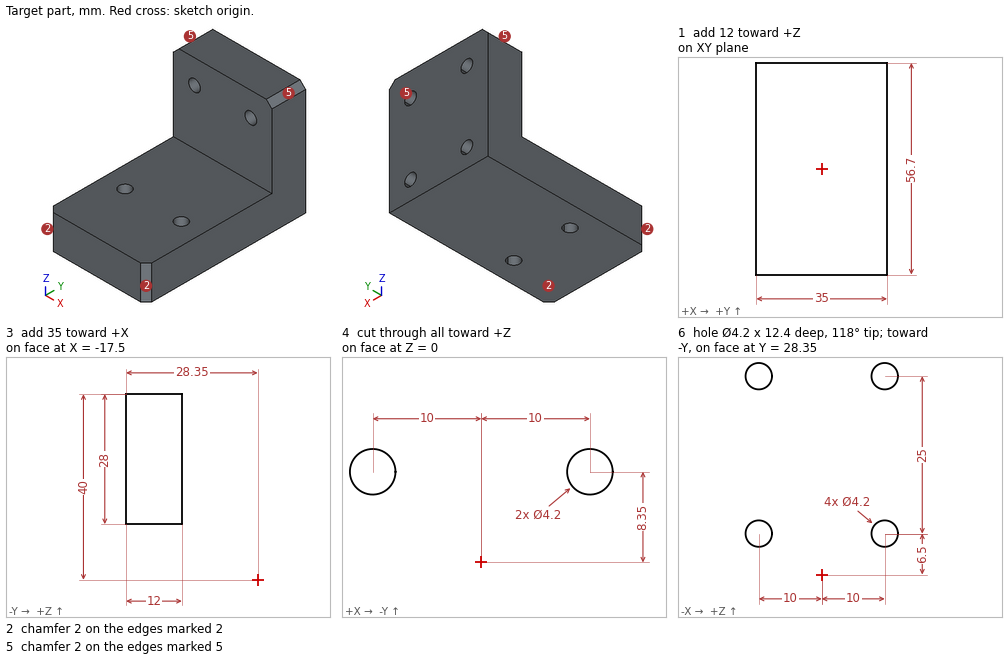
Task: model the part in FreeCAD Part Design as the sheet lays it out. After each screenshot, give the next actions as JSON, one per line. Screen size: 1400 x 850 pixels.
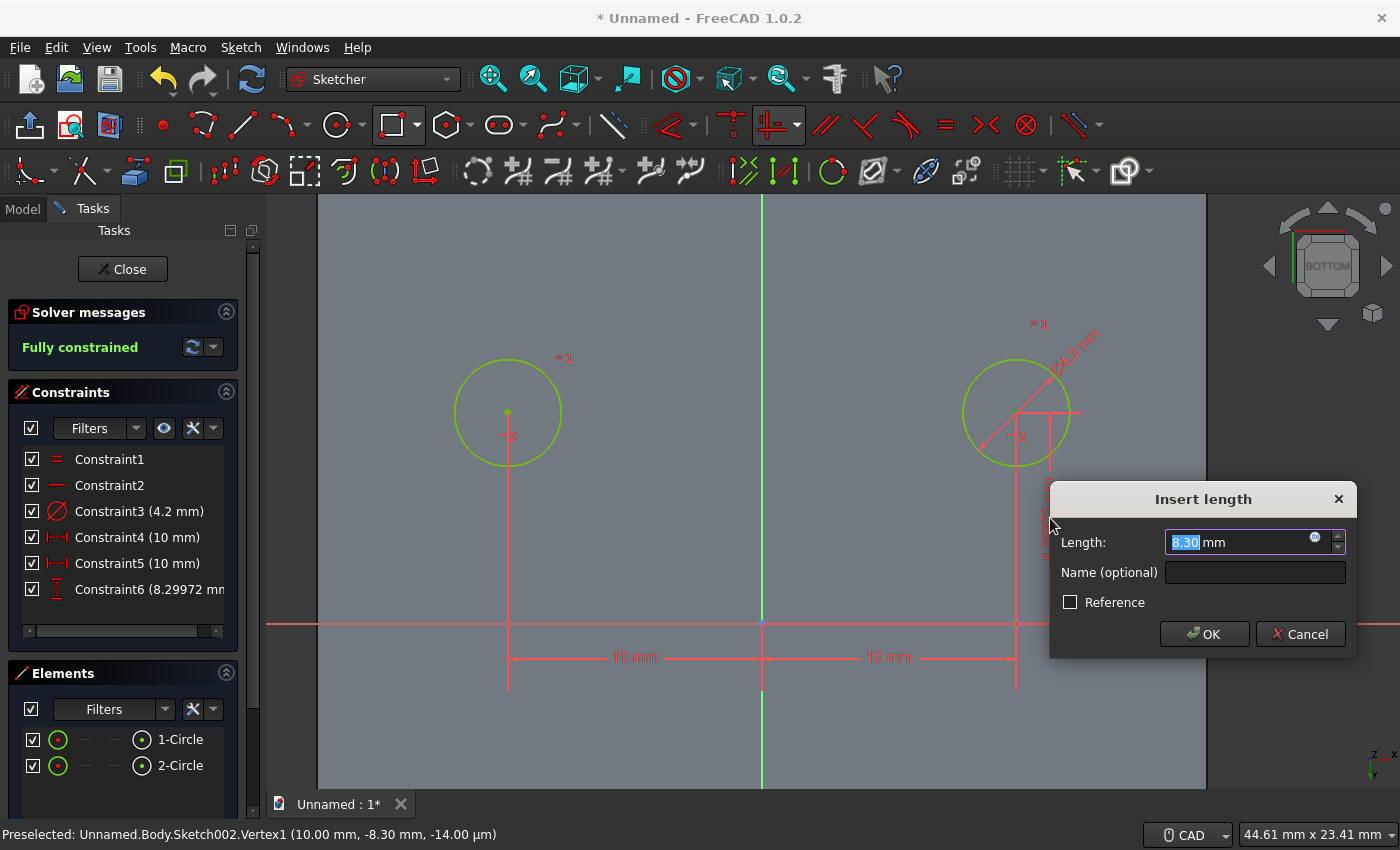
{"action": "type", "text": "8.35"}
{"action": "key", "text": "Return"}
{"action": "key", "text": "Escape"}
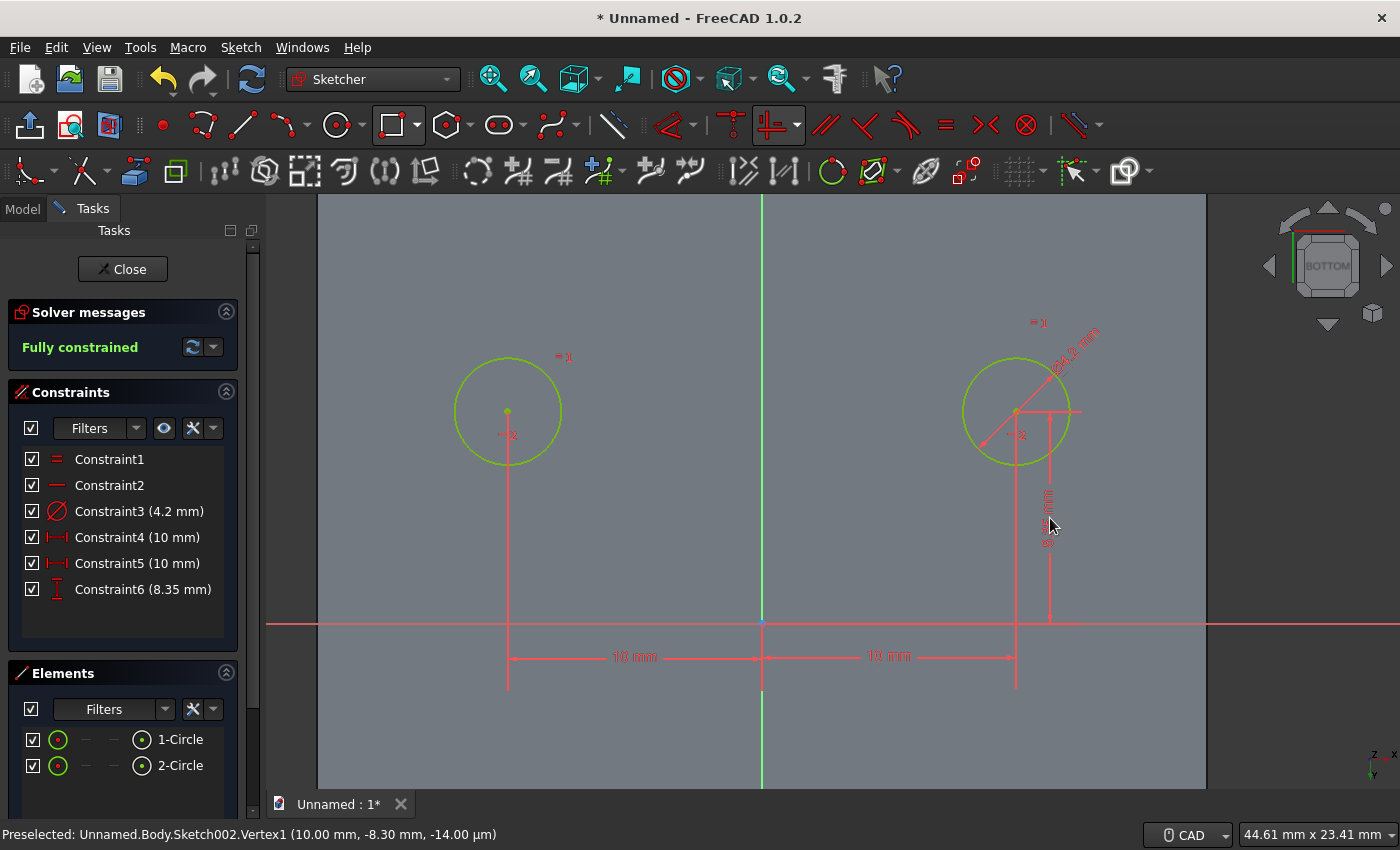
{"action": "left_click", "coordinate": [123, 269]}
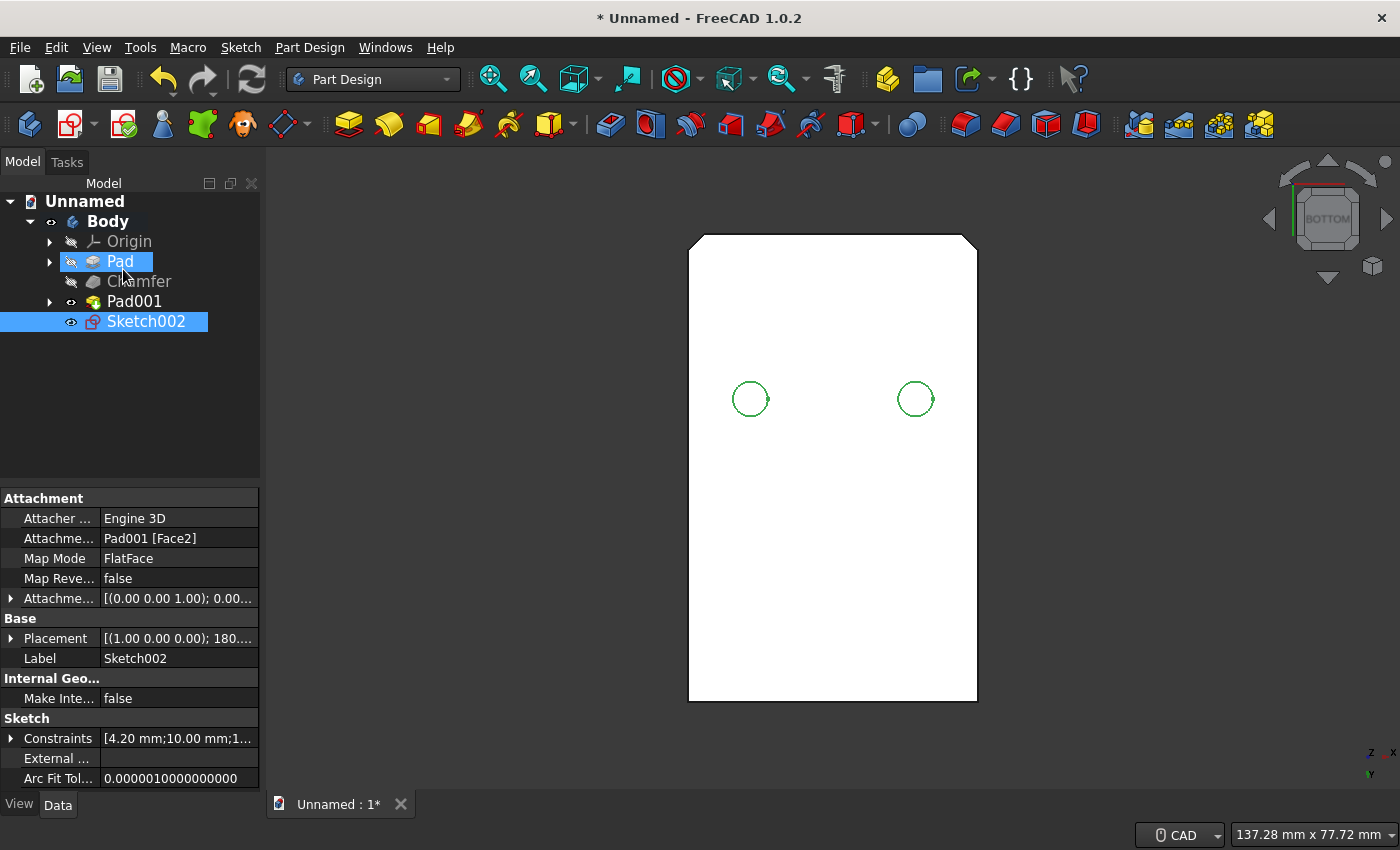
{"action": "left_click", "coordinate": [612, 124]}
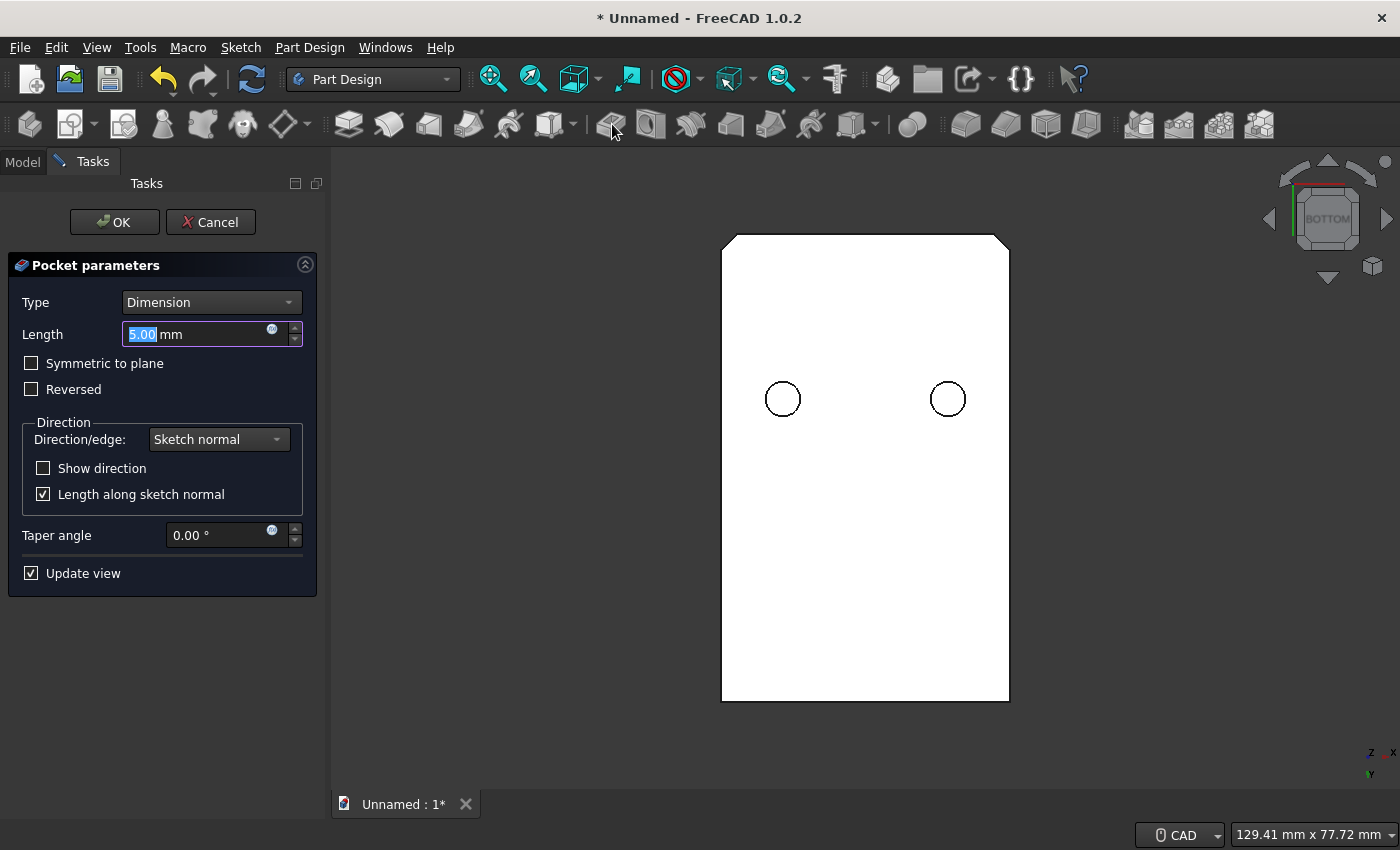
{"action": "left_click", "coordinate": [212, 302]}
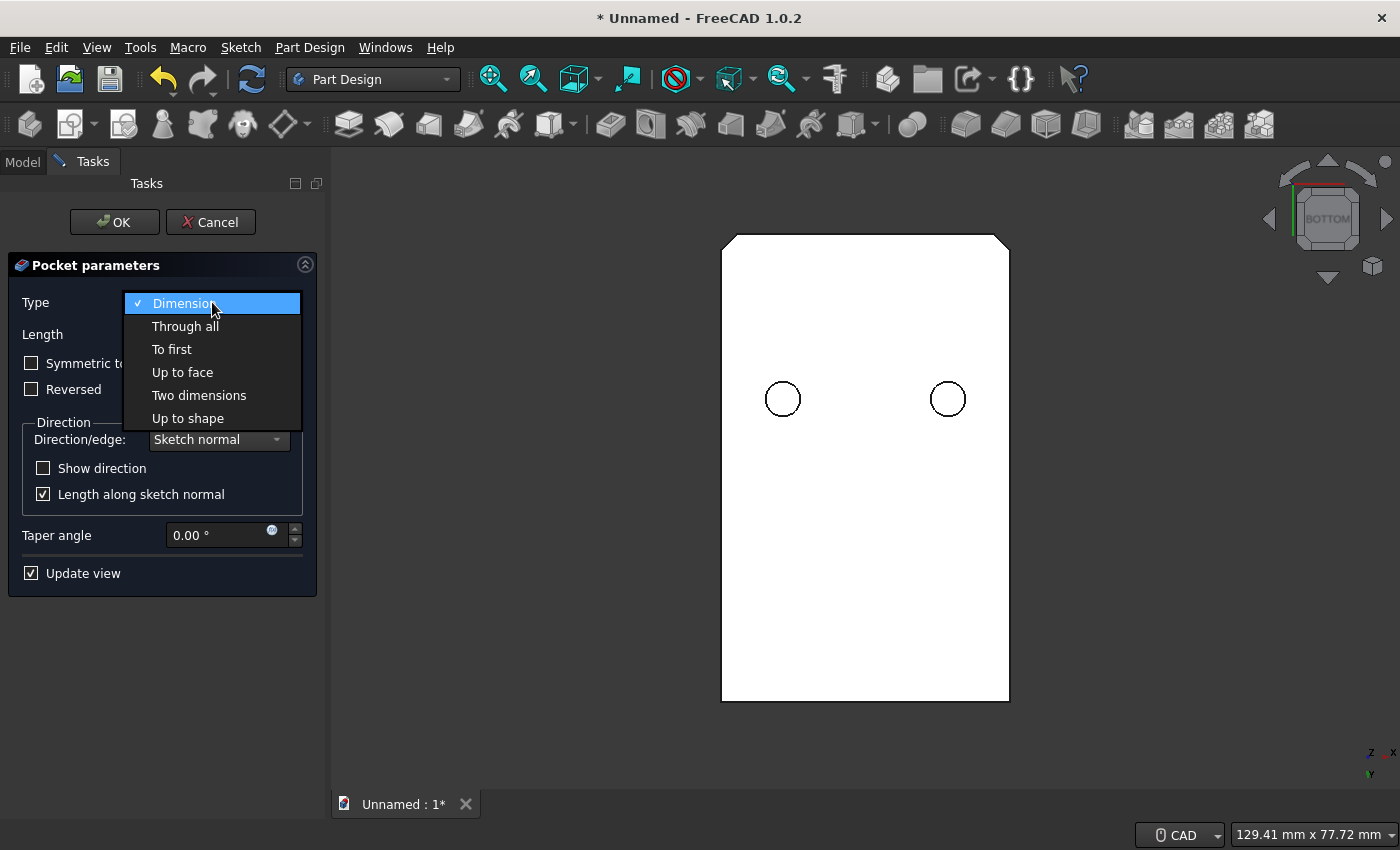
{"action": "left_click", "coordinate": [212, 326]}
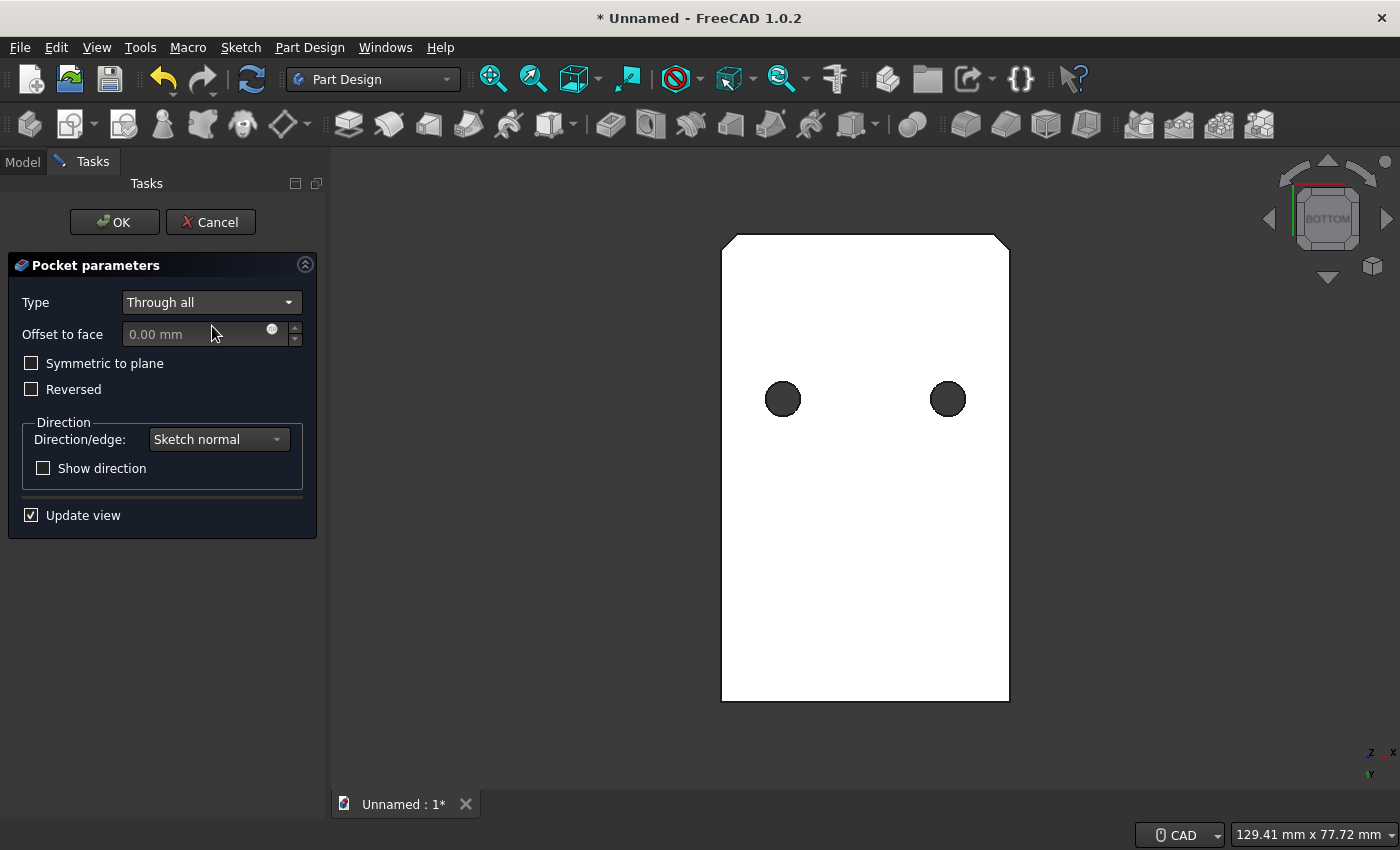
{"action": "left_click", "coordinate": [115, 222]}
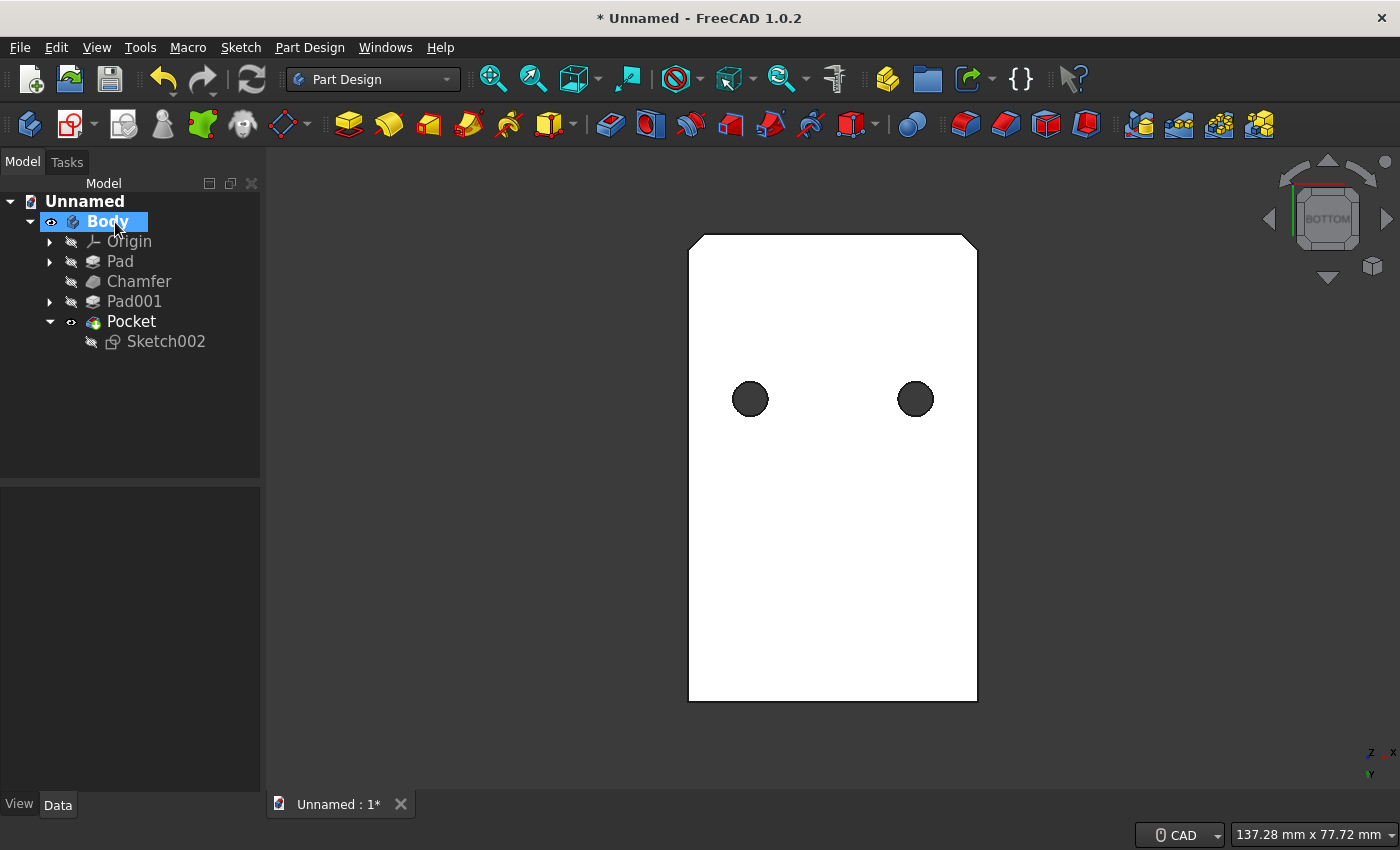
{"action": "key", "text": "0"}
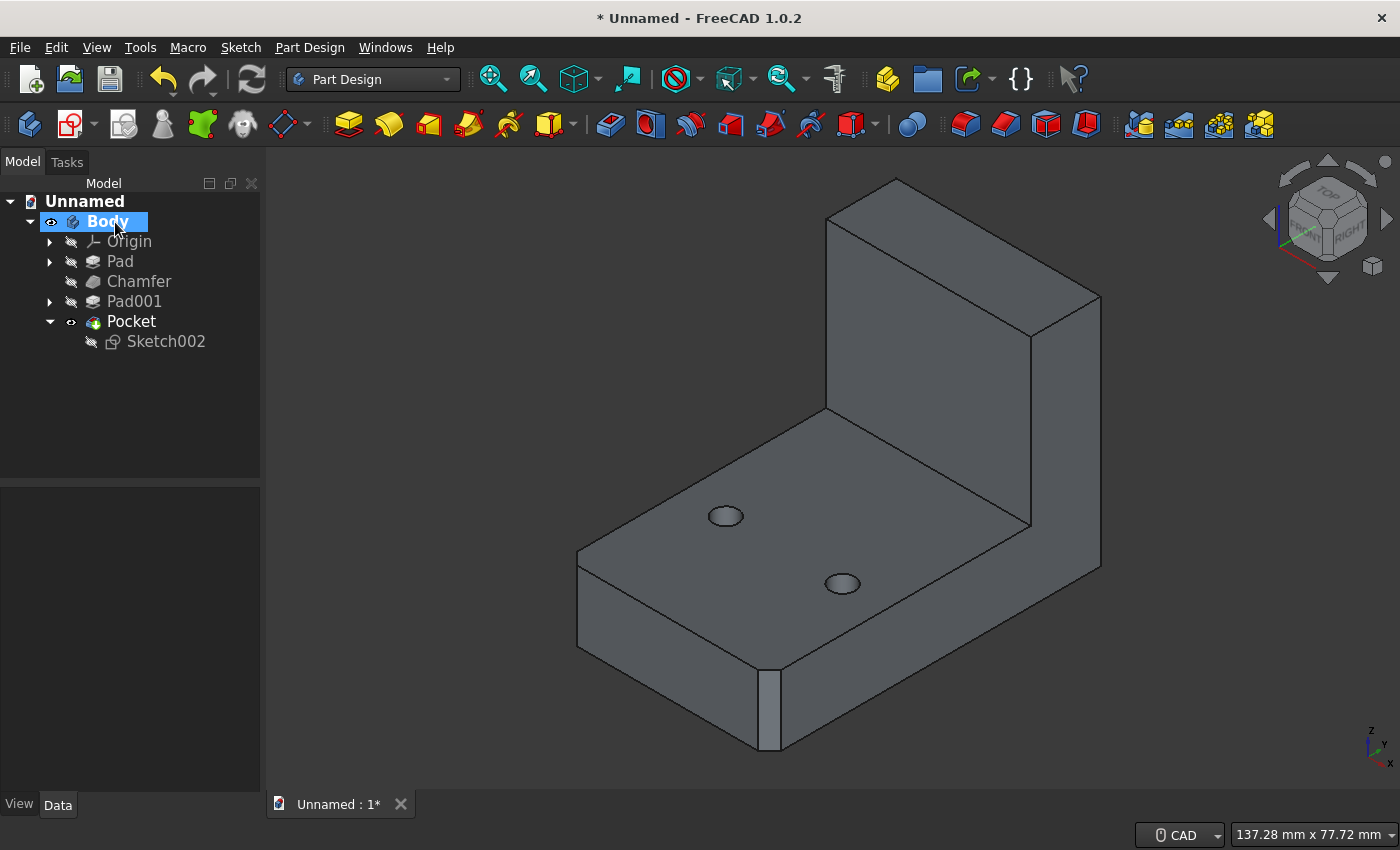
{"action": "left_click", "coordinate": [1066, 316]}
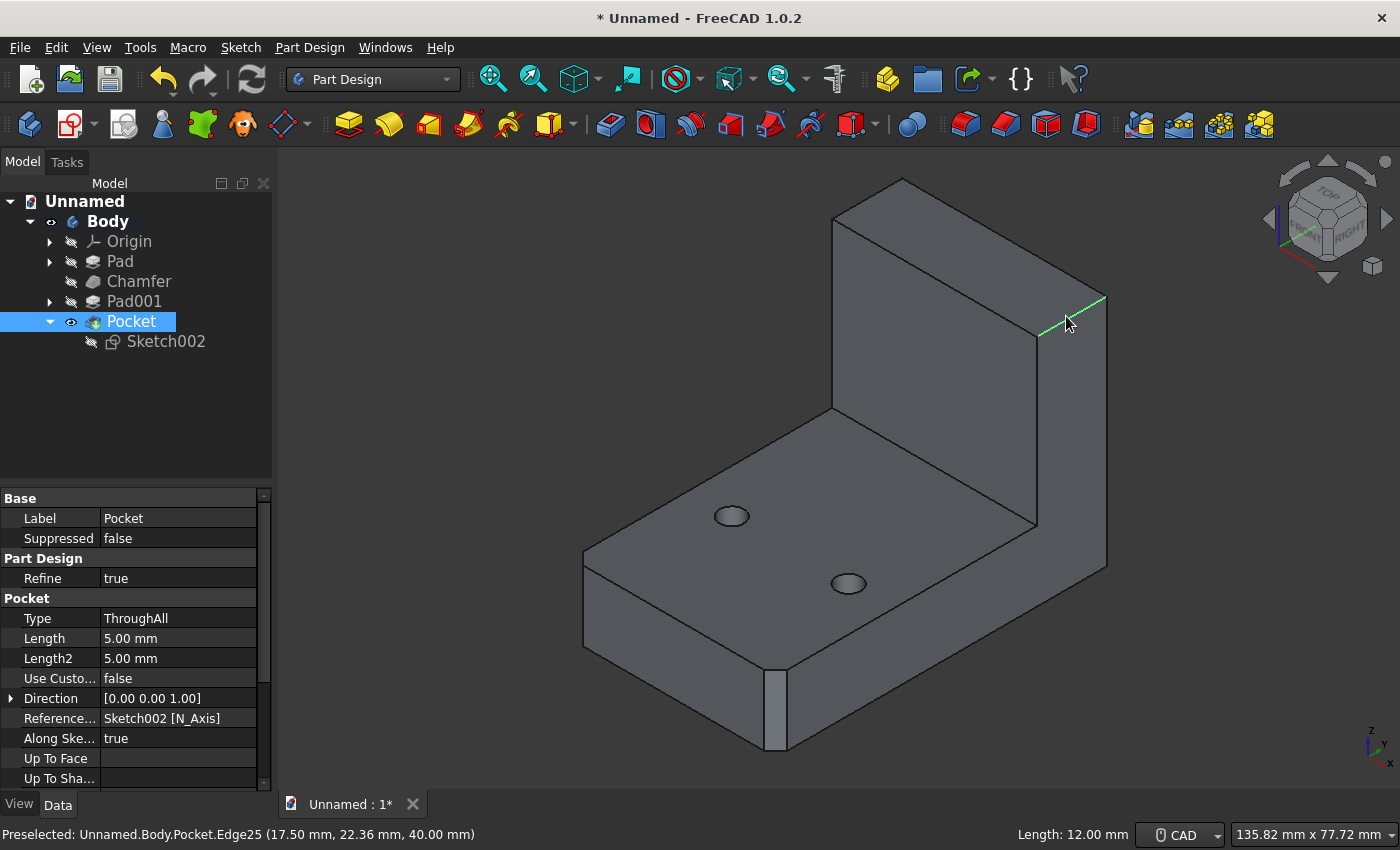
{"action": "key", "text": "2"}